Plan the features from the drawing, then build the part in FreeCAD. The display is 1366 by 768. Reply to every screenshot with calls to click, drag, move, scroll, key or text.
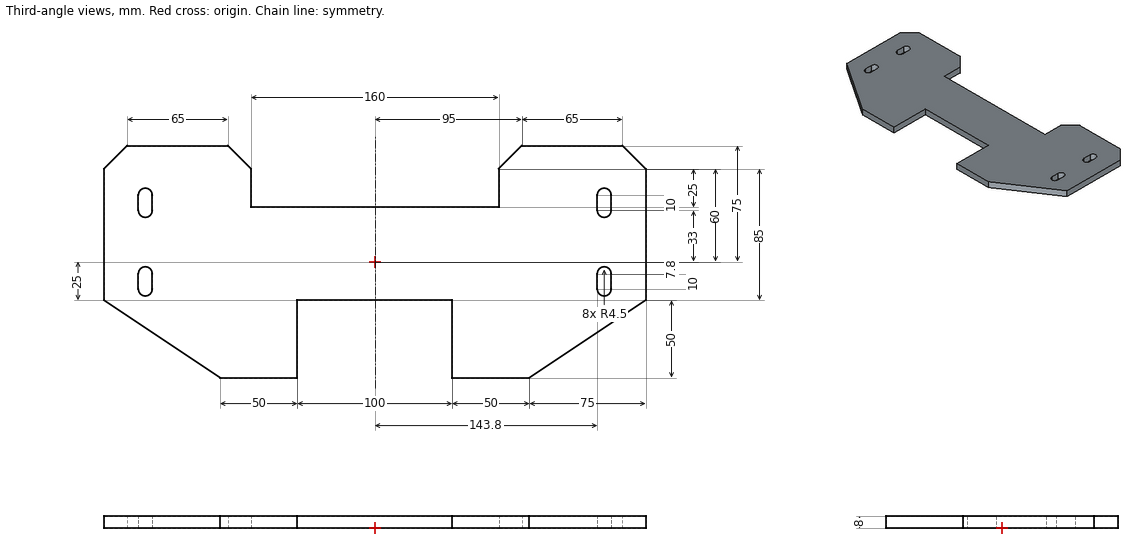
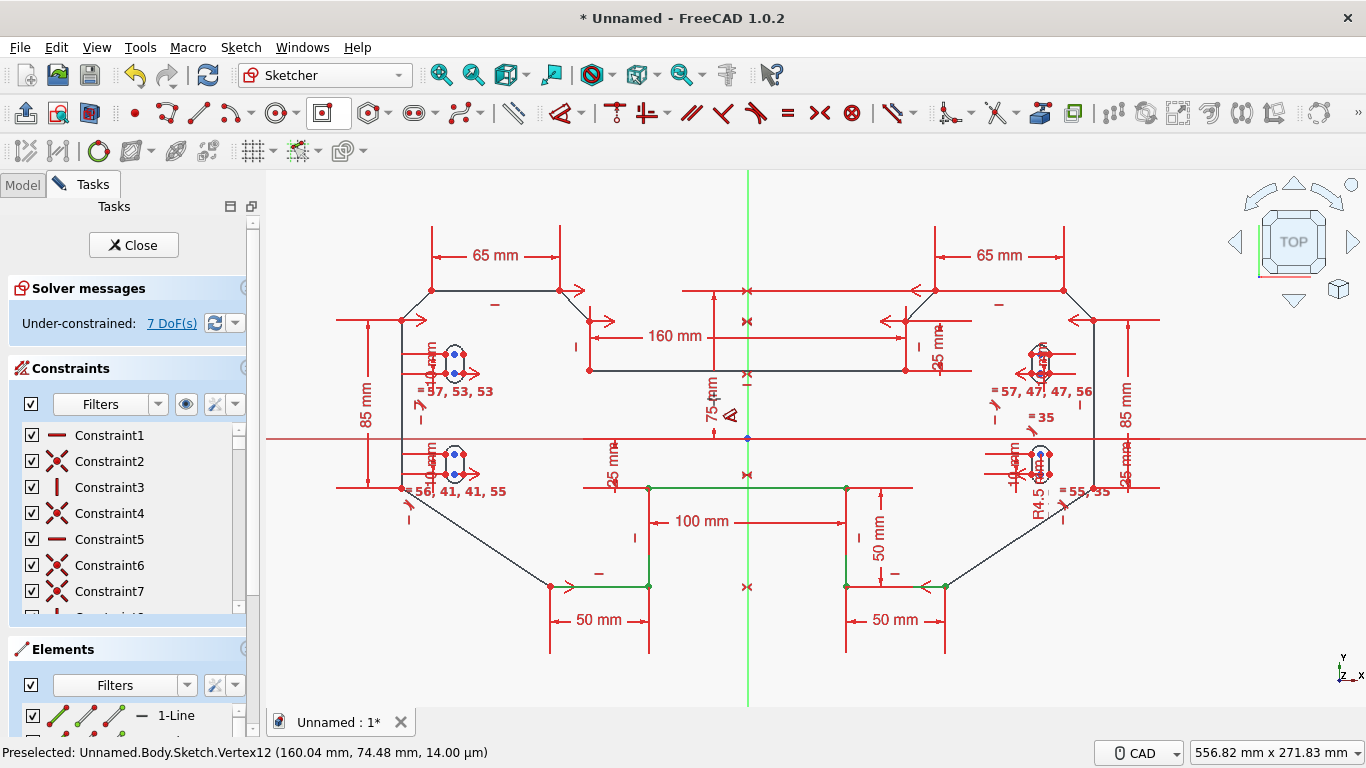
click(935, 291)
click(842, 257)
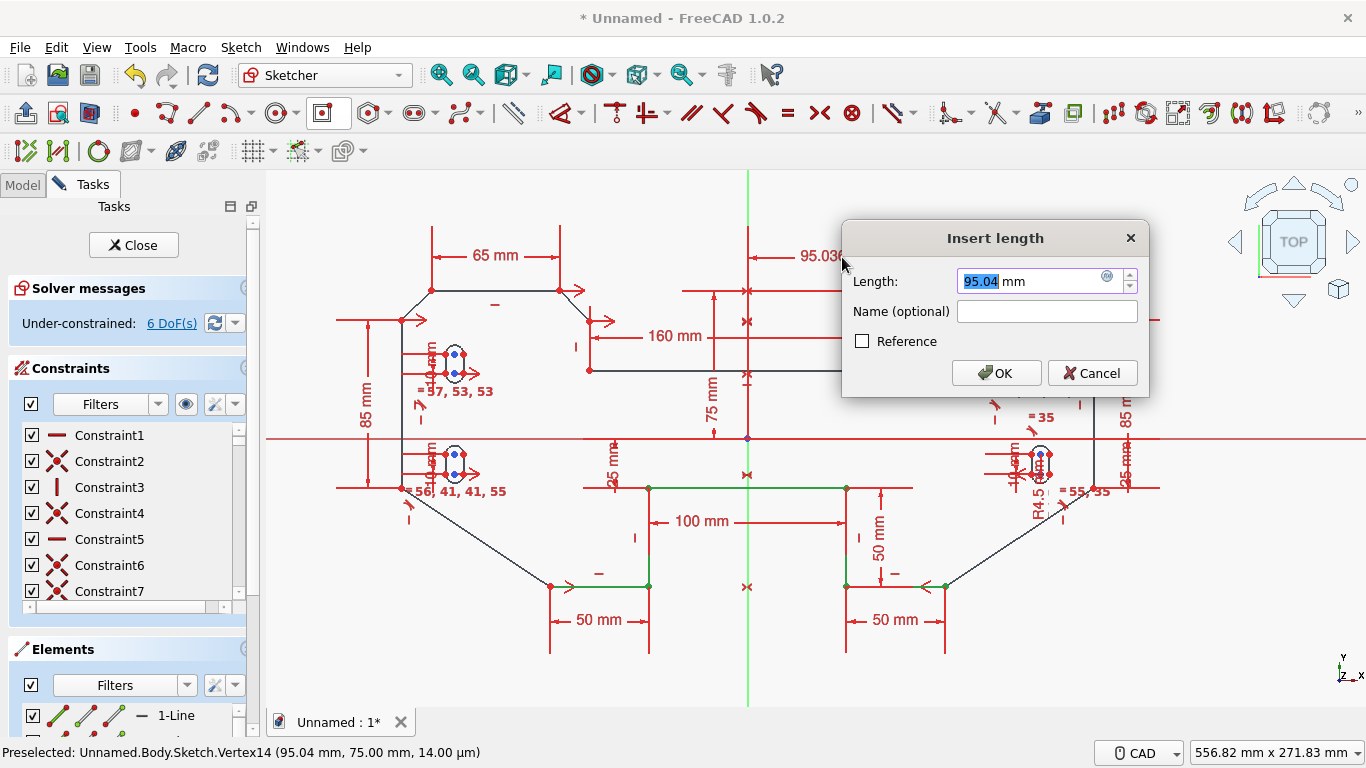
text(95)
key(Return)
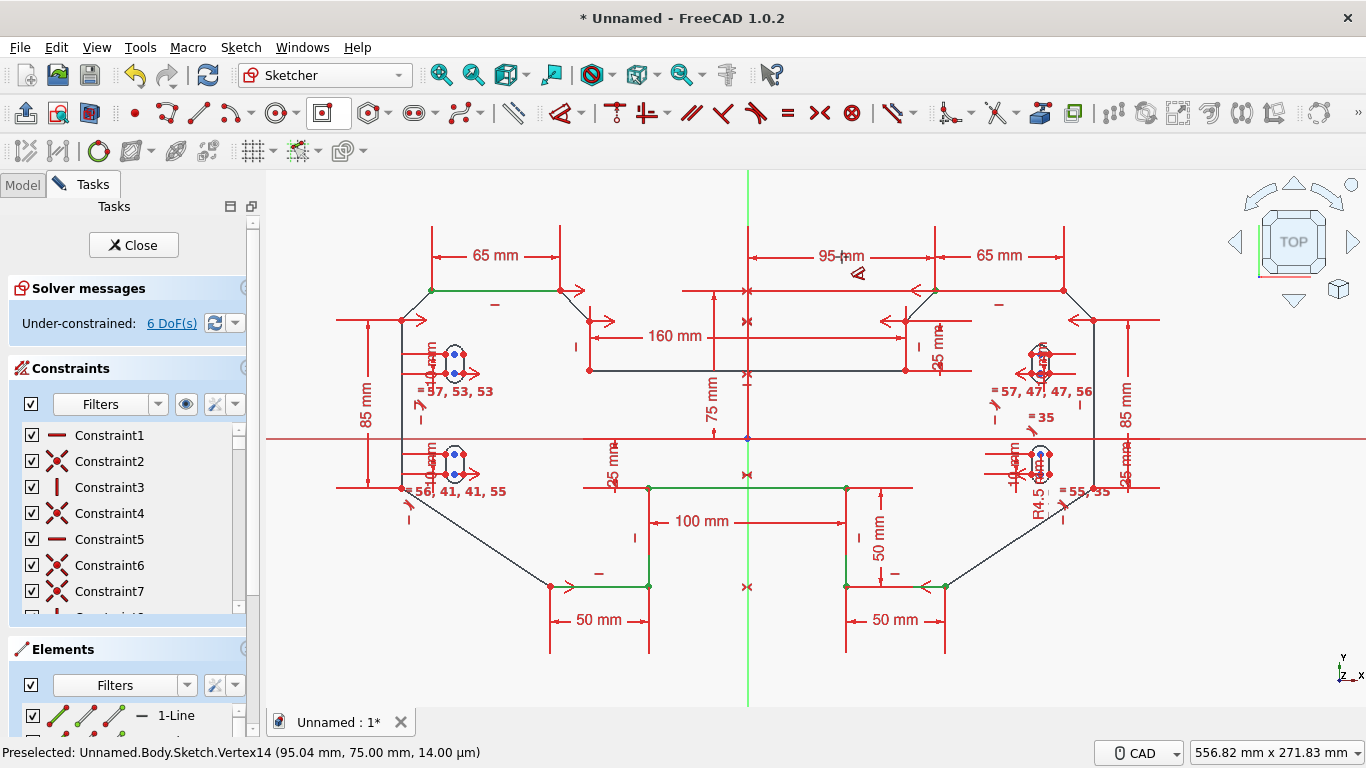
click(906, 321)
click(940, 380)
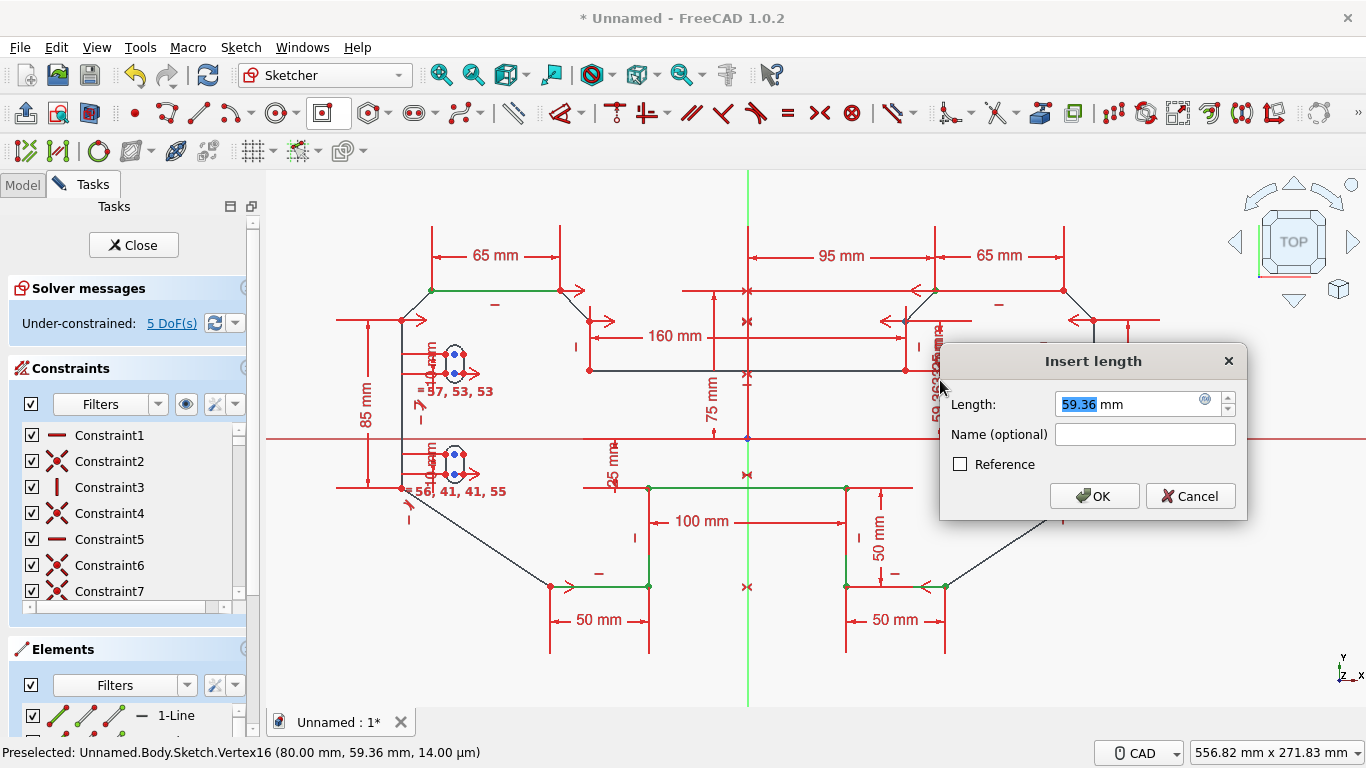
text(60)
key(Return)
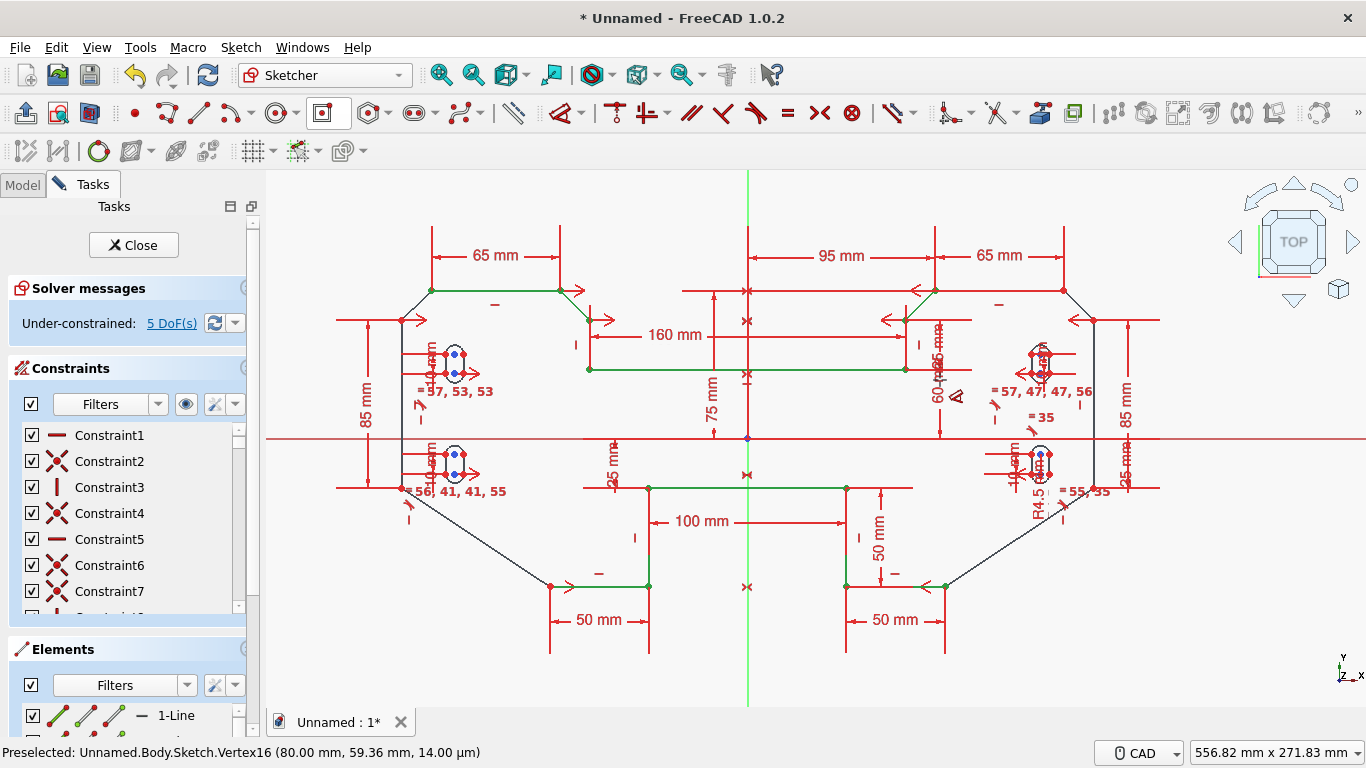
scroll(1032, 374, up, 2)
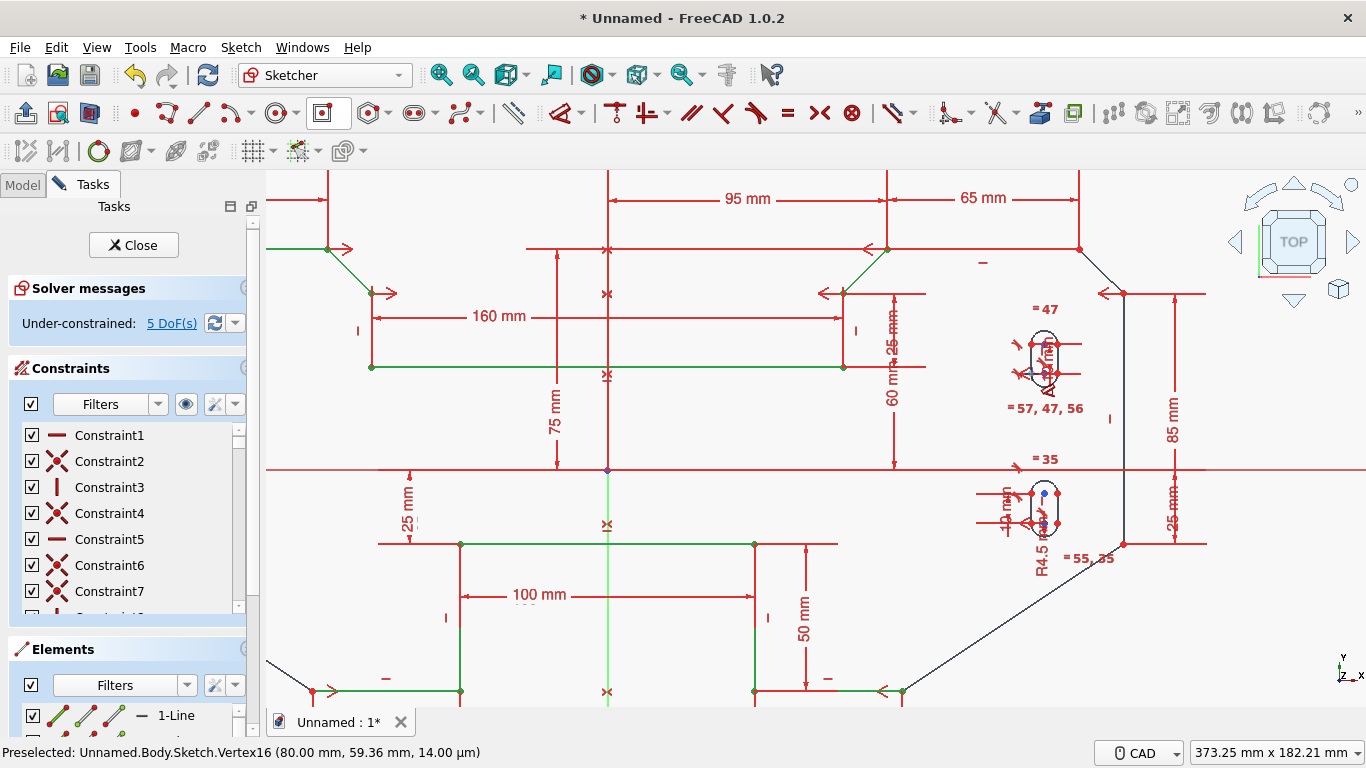
click(1031, 374)
click(1065, 422)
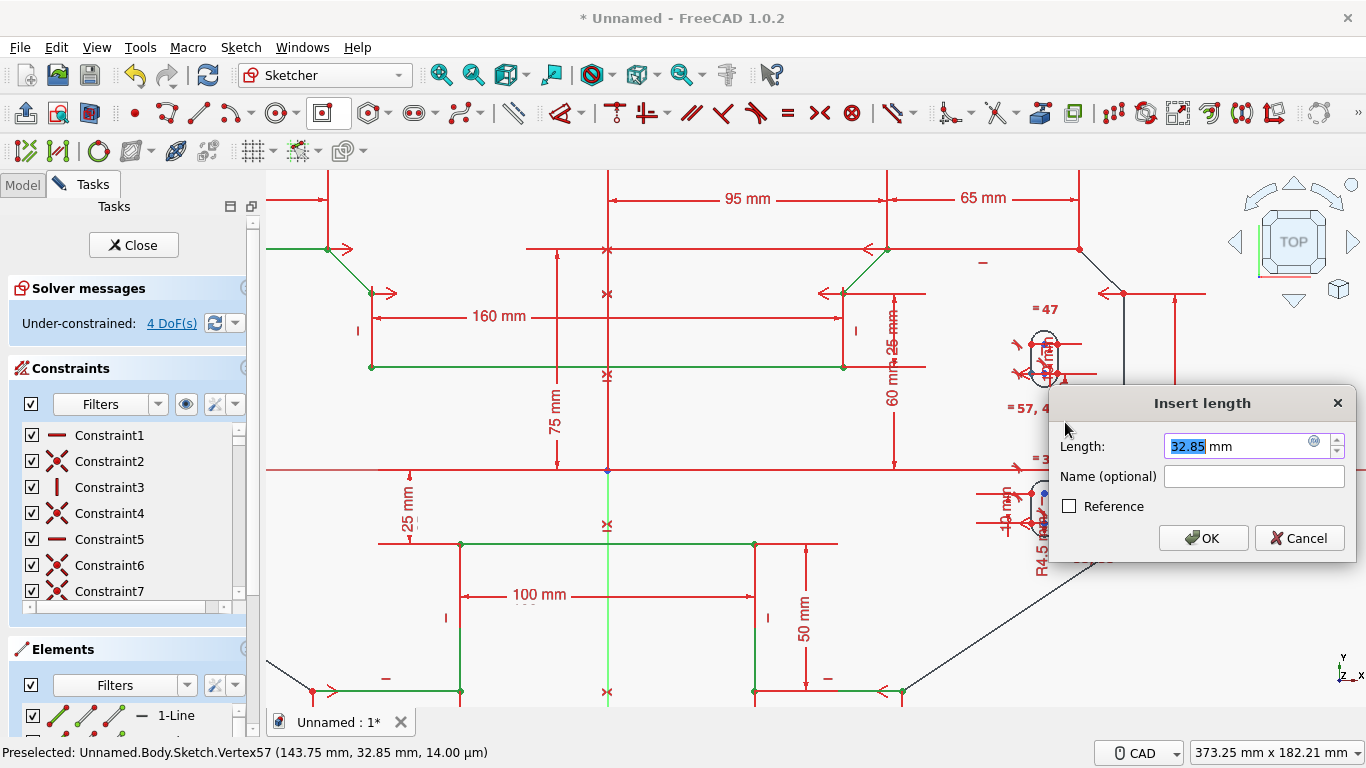
text(33)
key(Return)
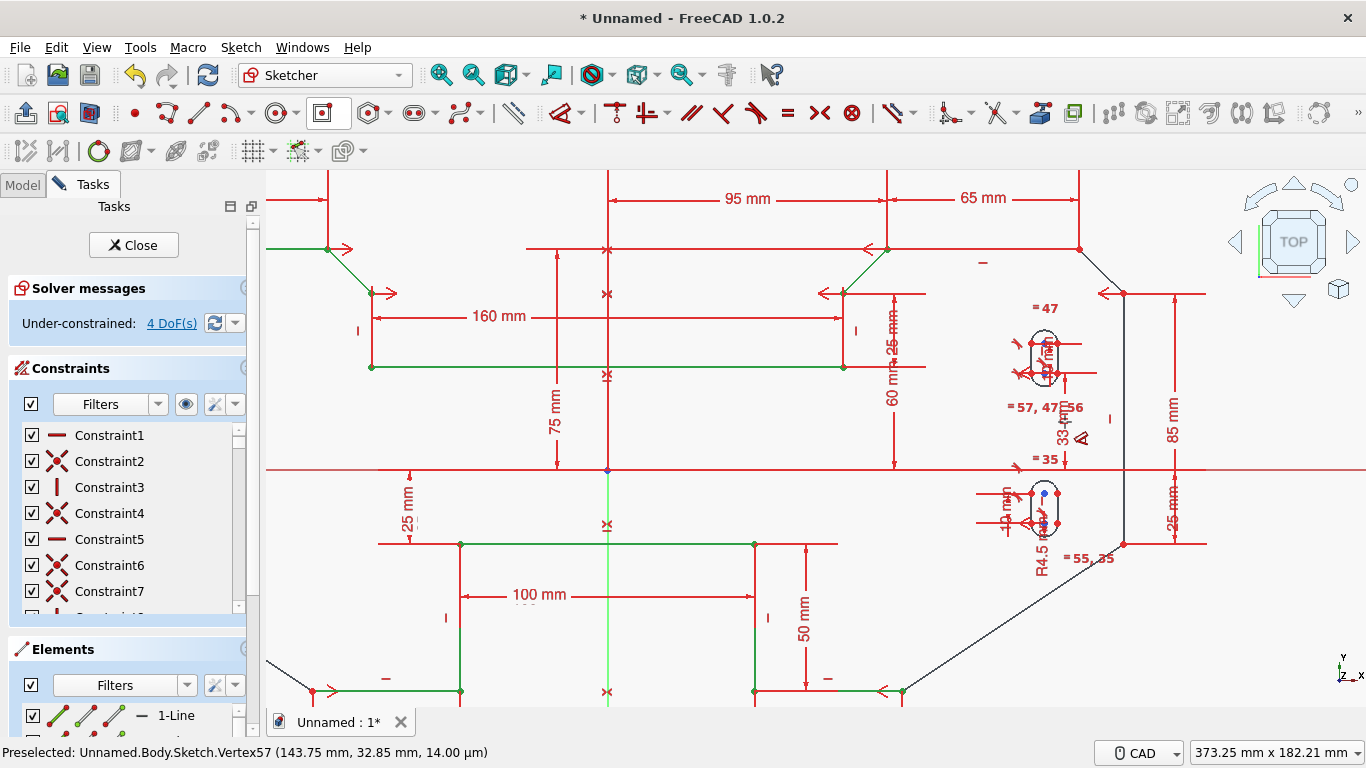
click(969, 647)
click(935, 510)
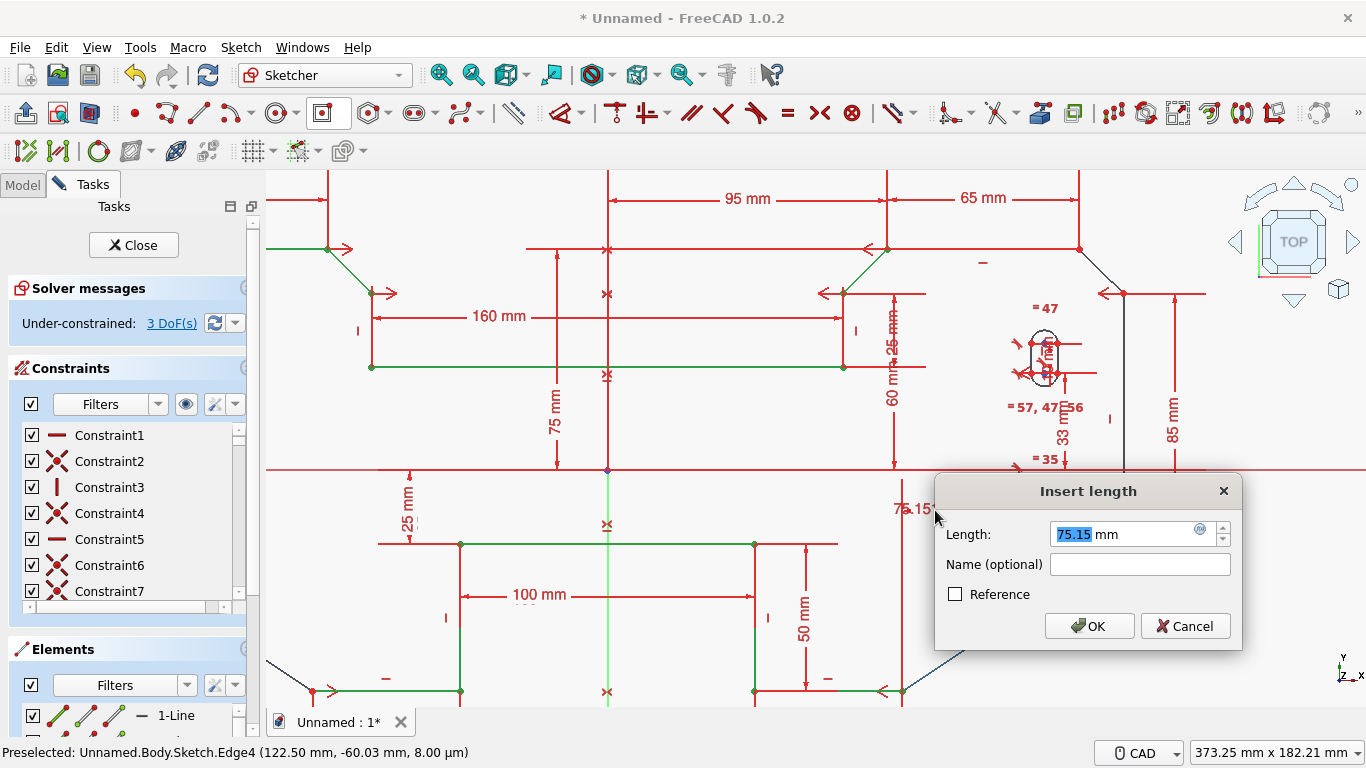
text(75)
key(Return)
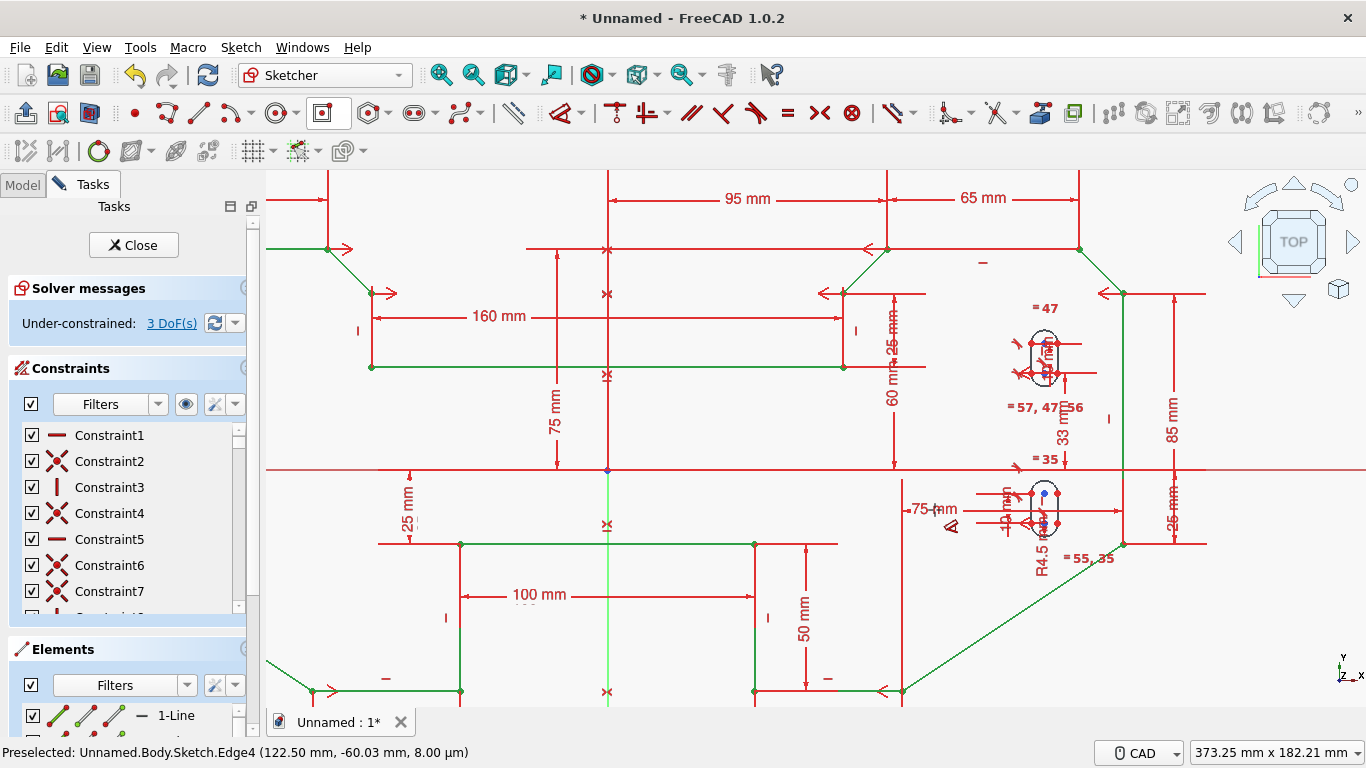
scroll(1058, 494, up, 3)